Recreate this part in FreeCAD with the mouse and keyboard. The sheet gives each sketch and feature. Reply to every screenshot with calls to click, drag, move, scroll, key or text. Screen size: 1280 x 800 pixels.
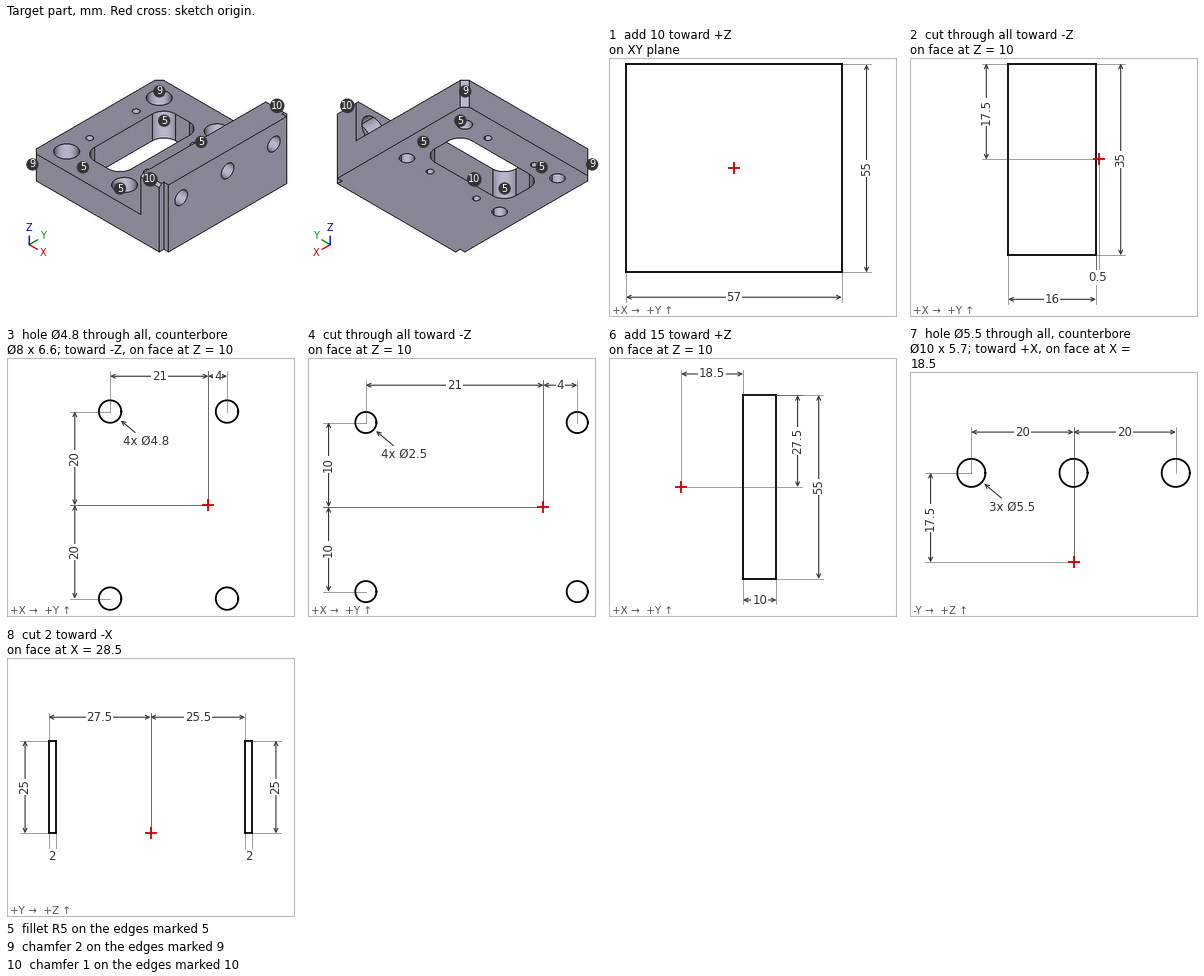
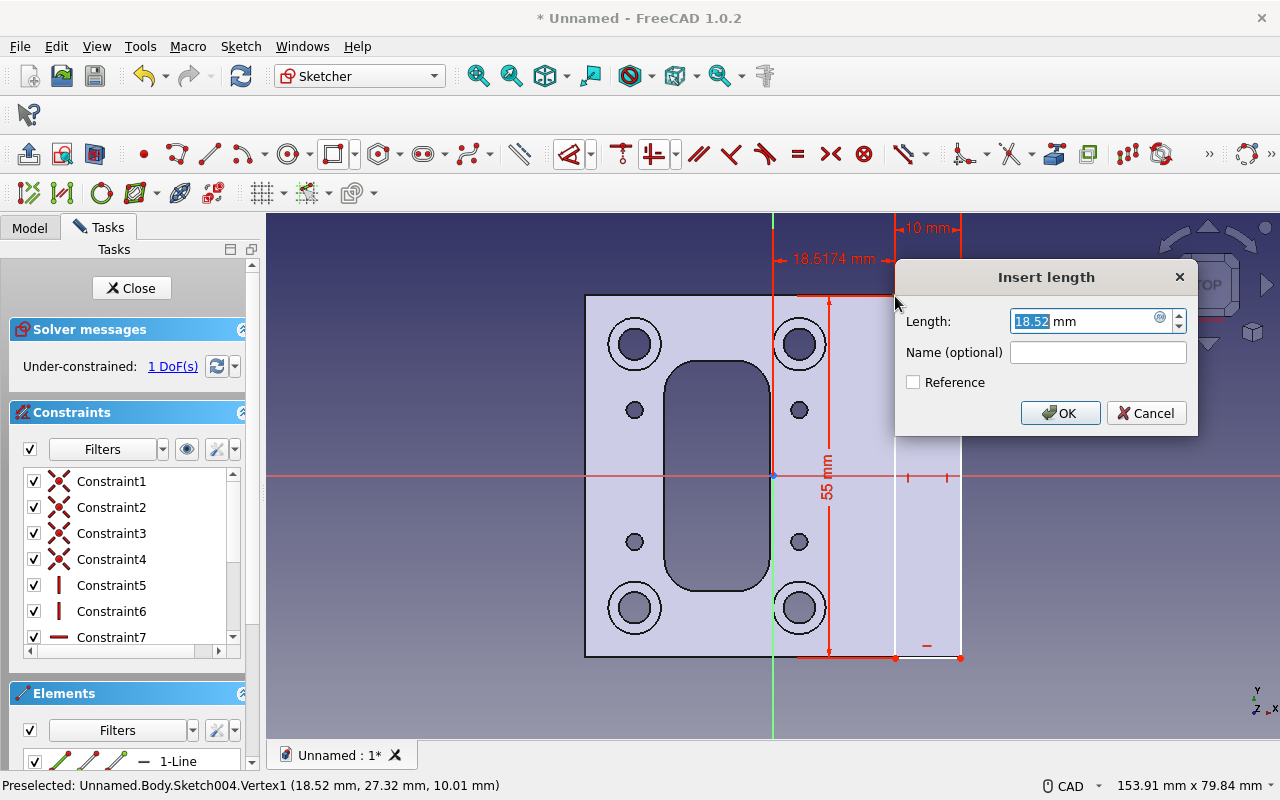
text(18.5)
key(Return)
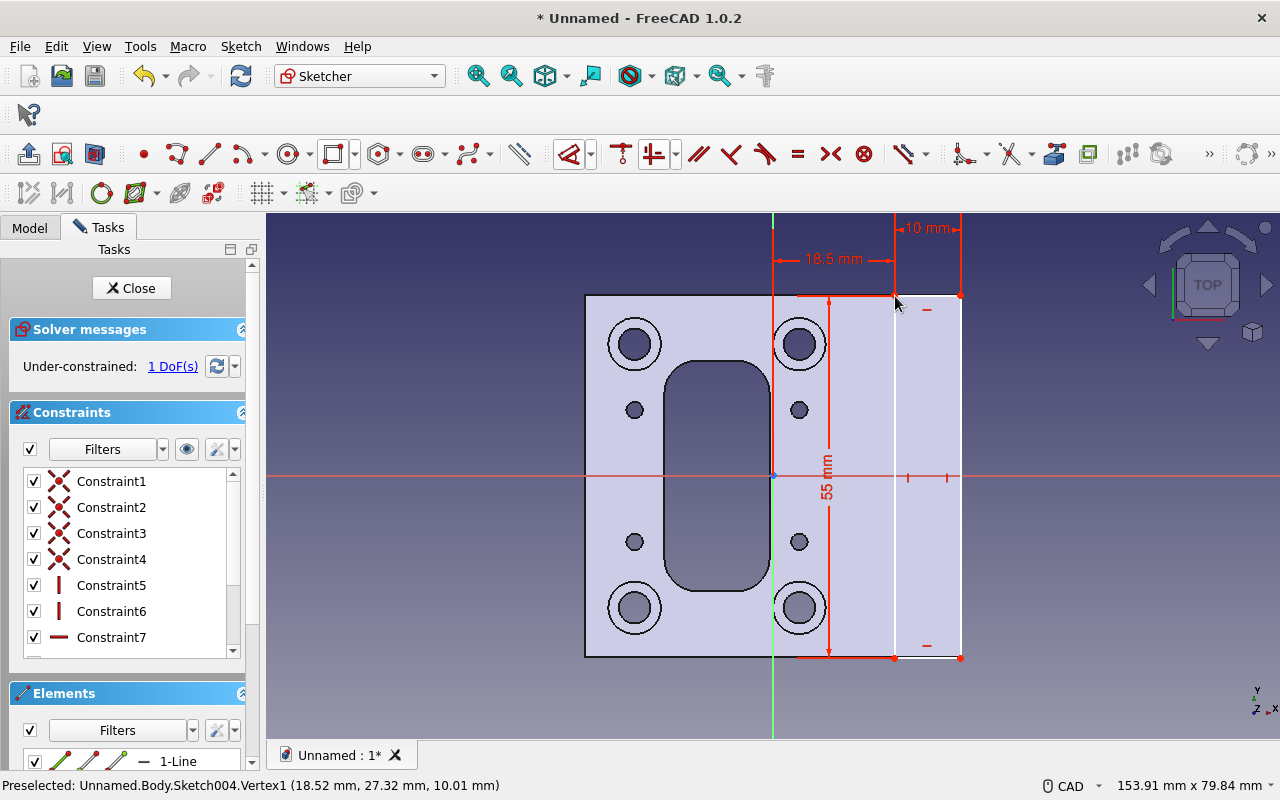
click(895, 296)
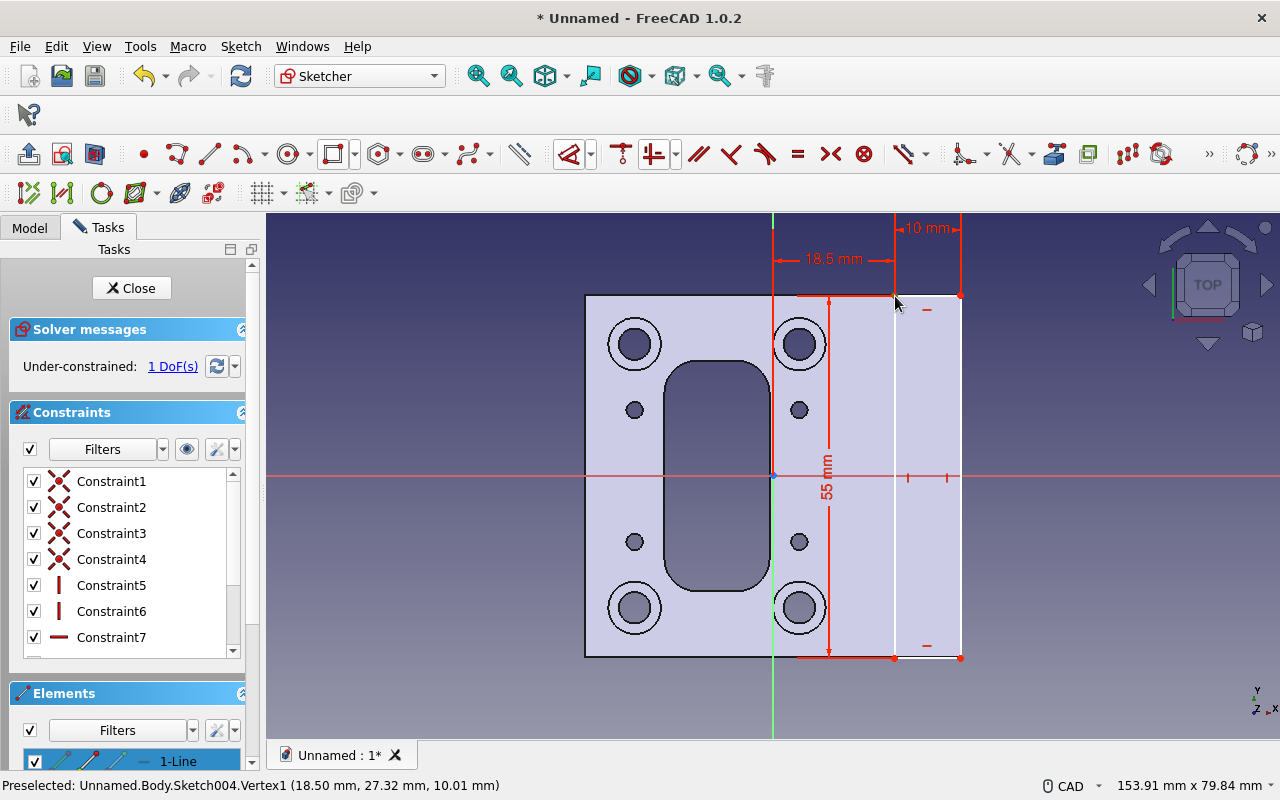
key(i)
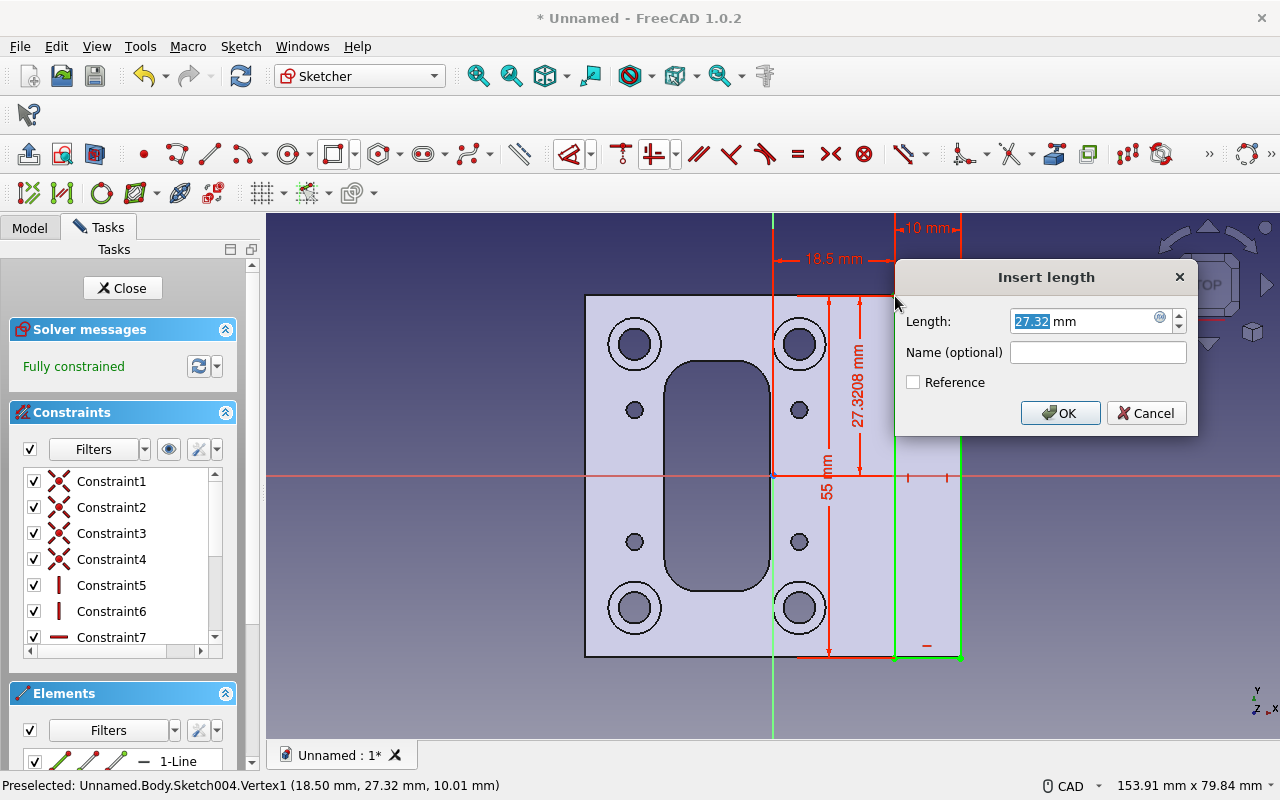
text(27.5)
key(Return)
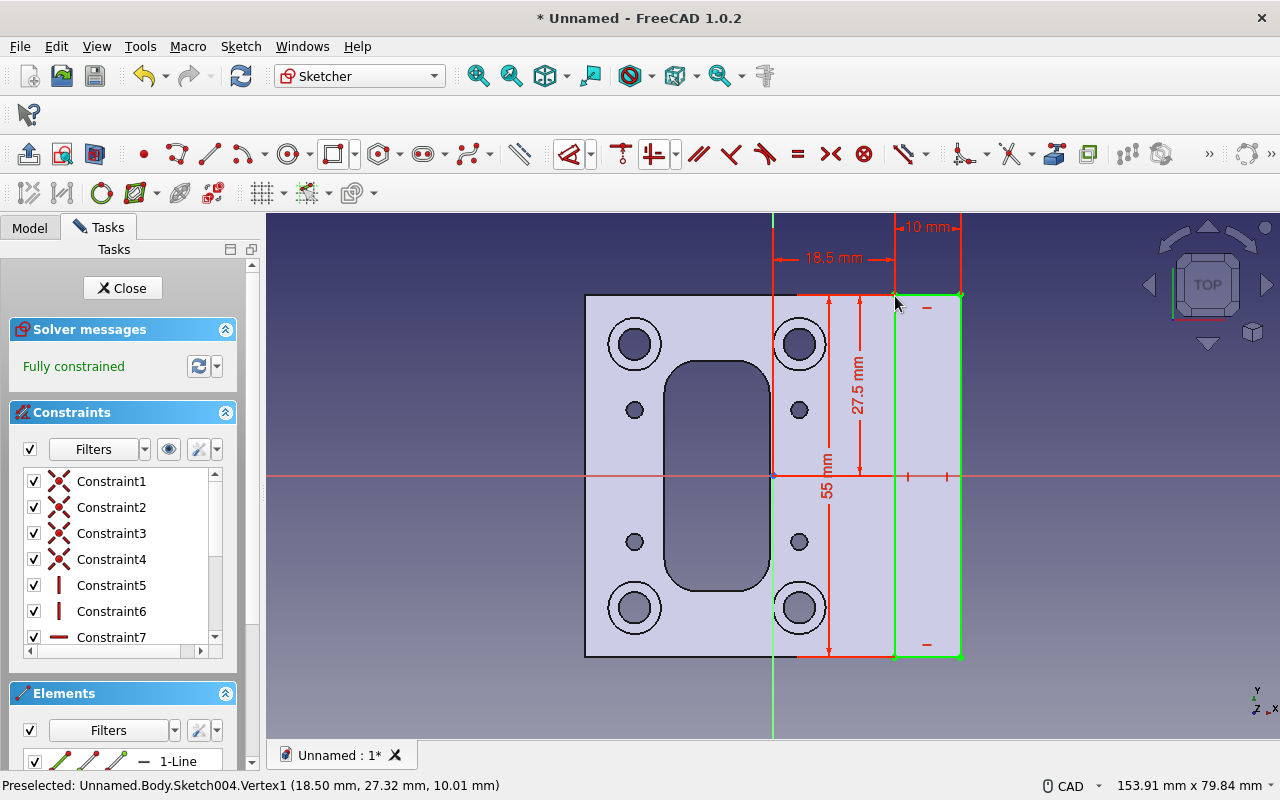
click(123, 288)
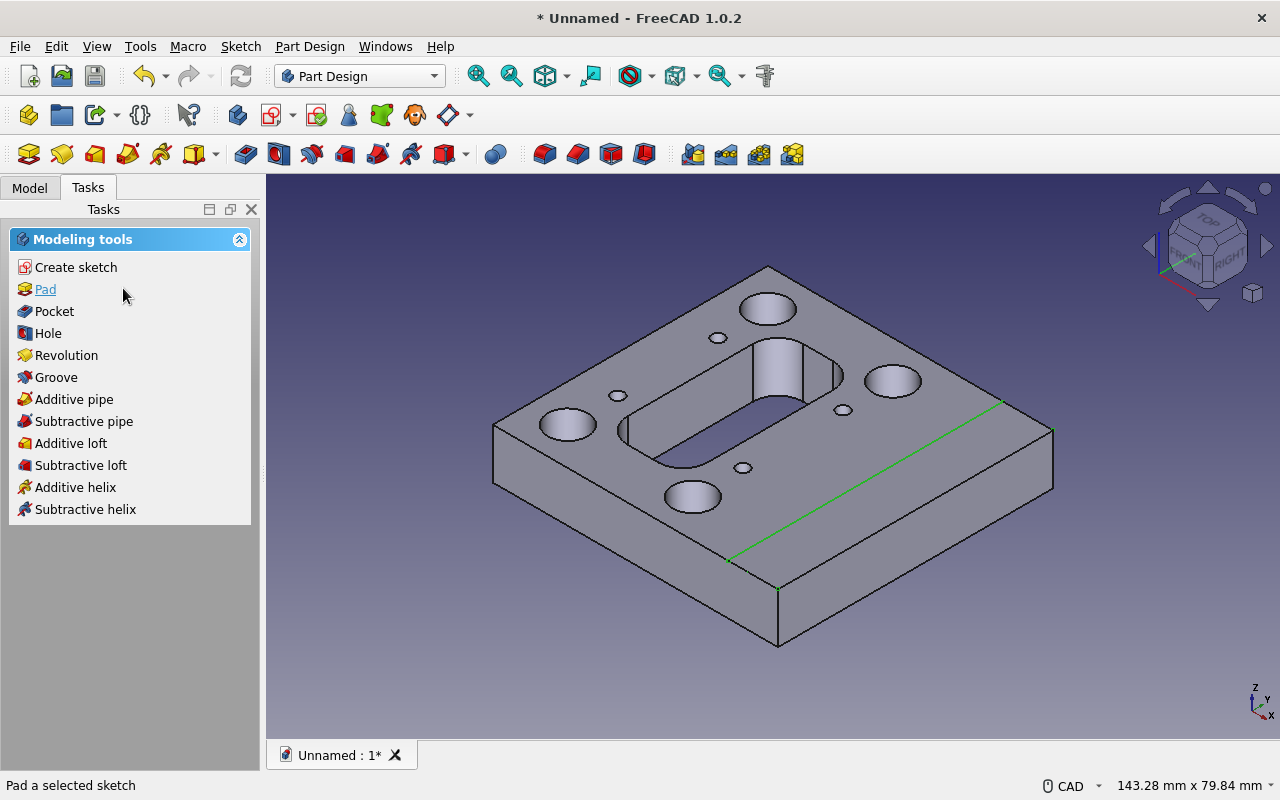
click(29, 154)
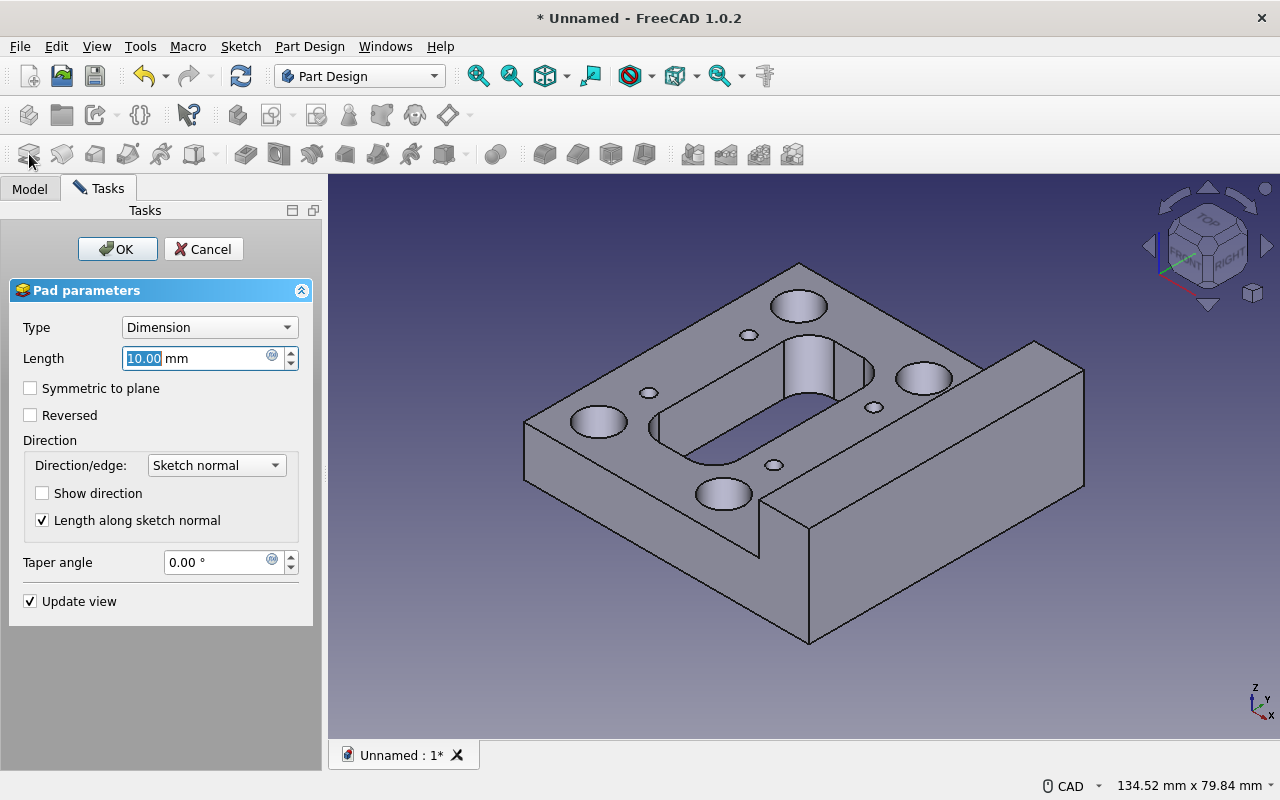
text(15)
key(Tab)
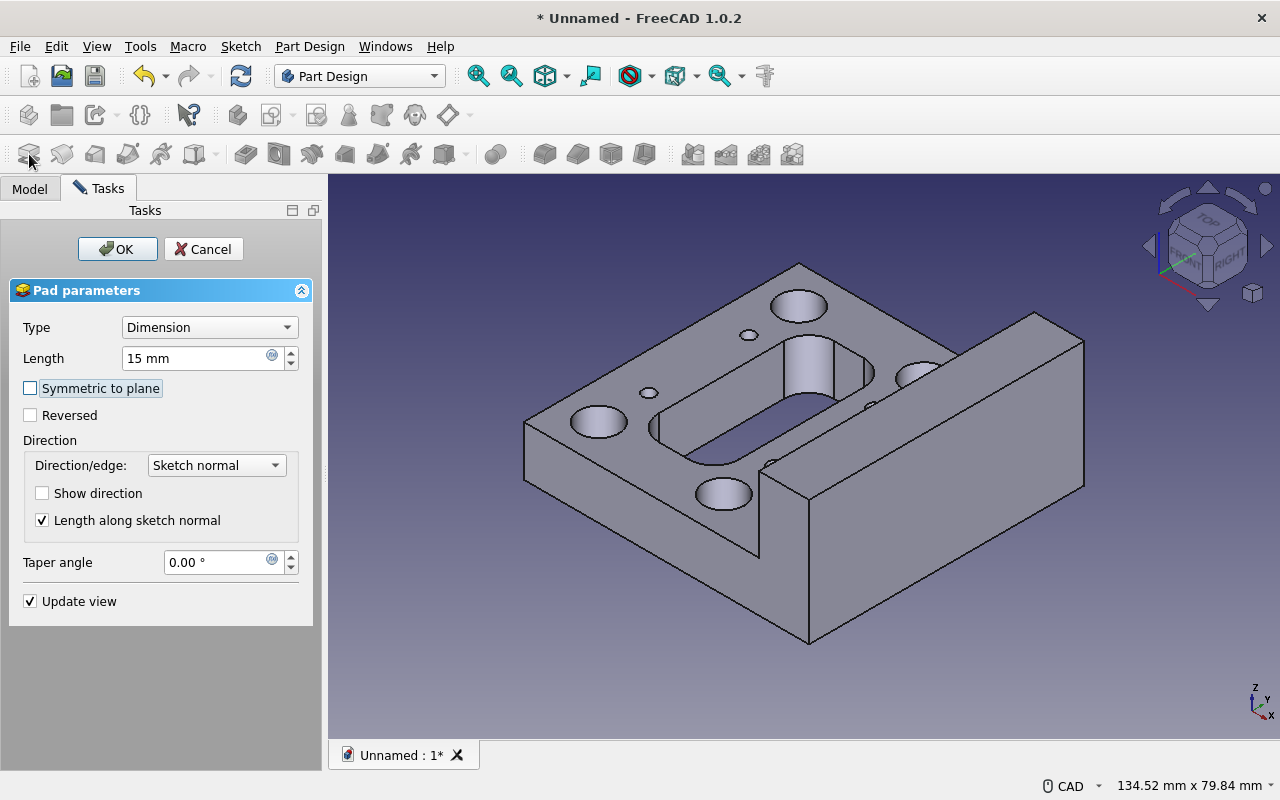
click(118, 249)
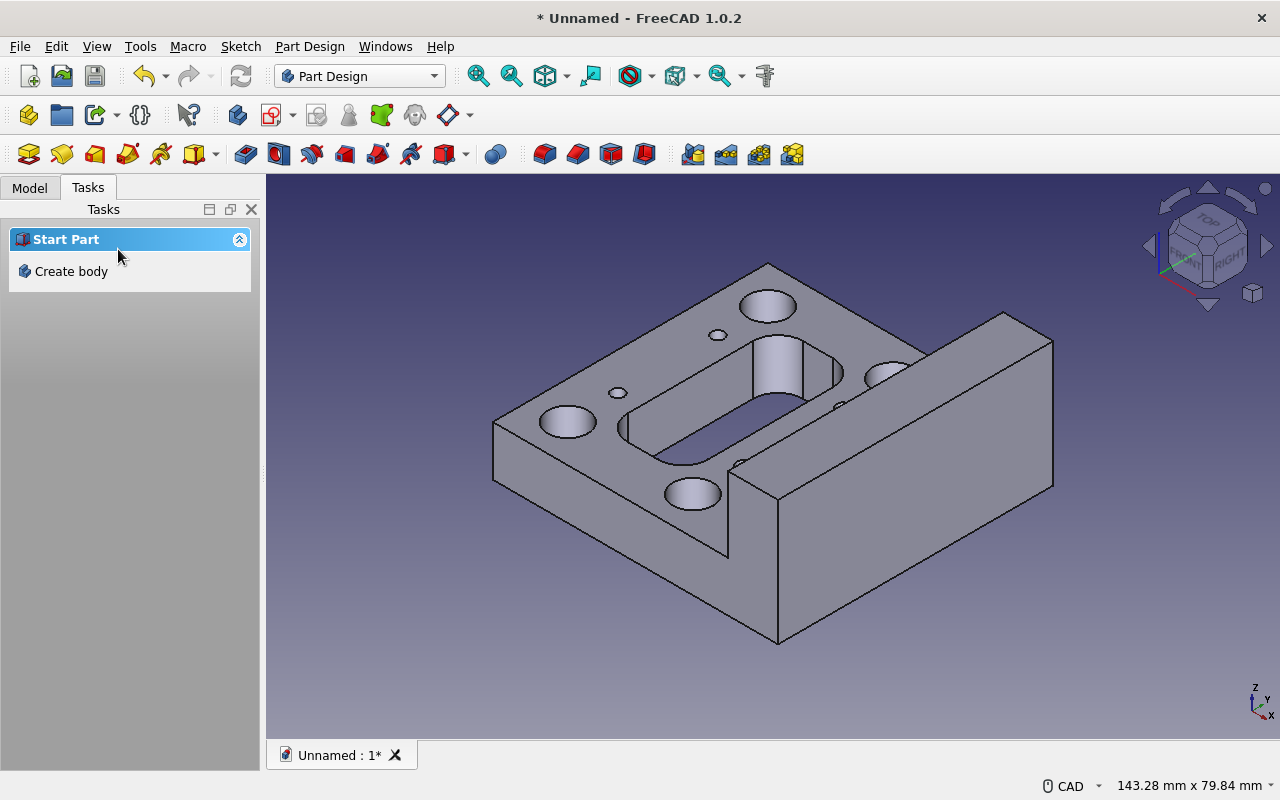
key(6)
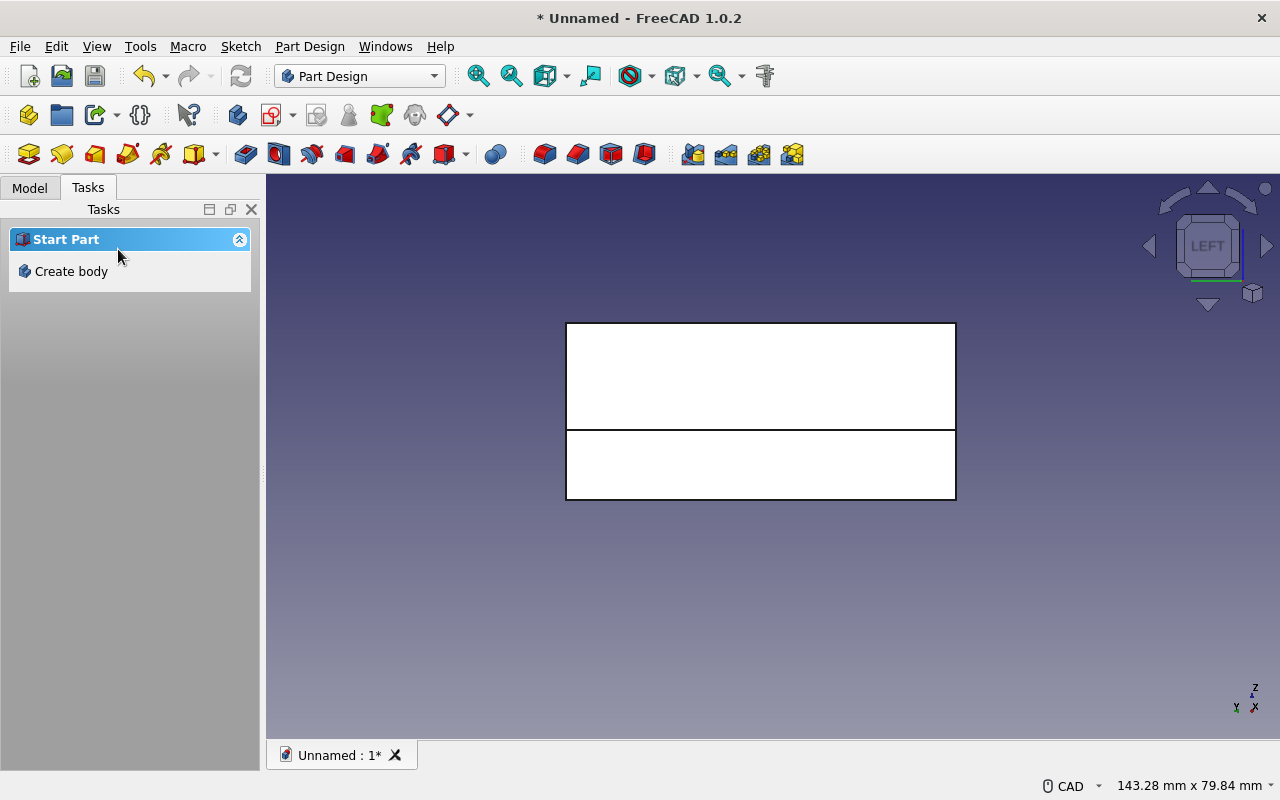
key(v)
key(f)